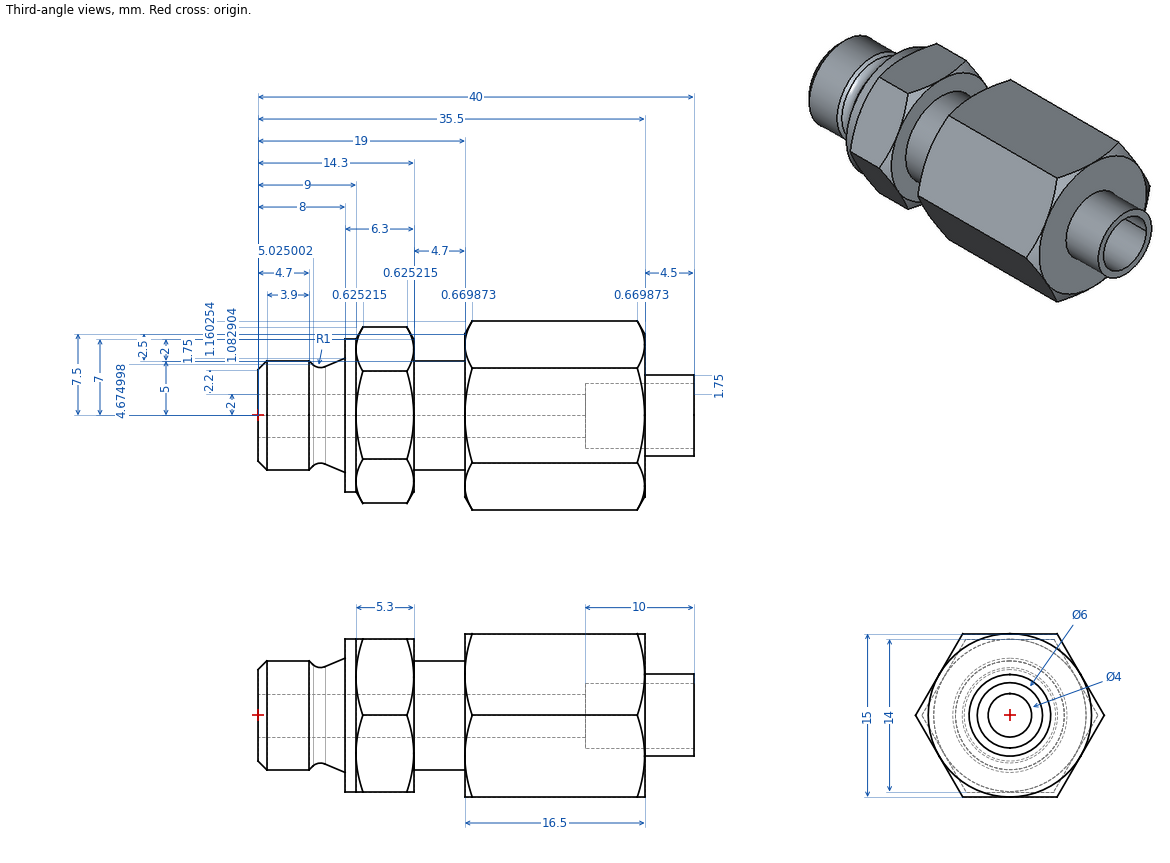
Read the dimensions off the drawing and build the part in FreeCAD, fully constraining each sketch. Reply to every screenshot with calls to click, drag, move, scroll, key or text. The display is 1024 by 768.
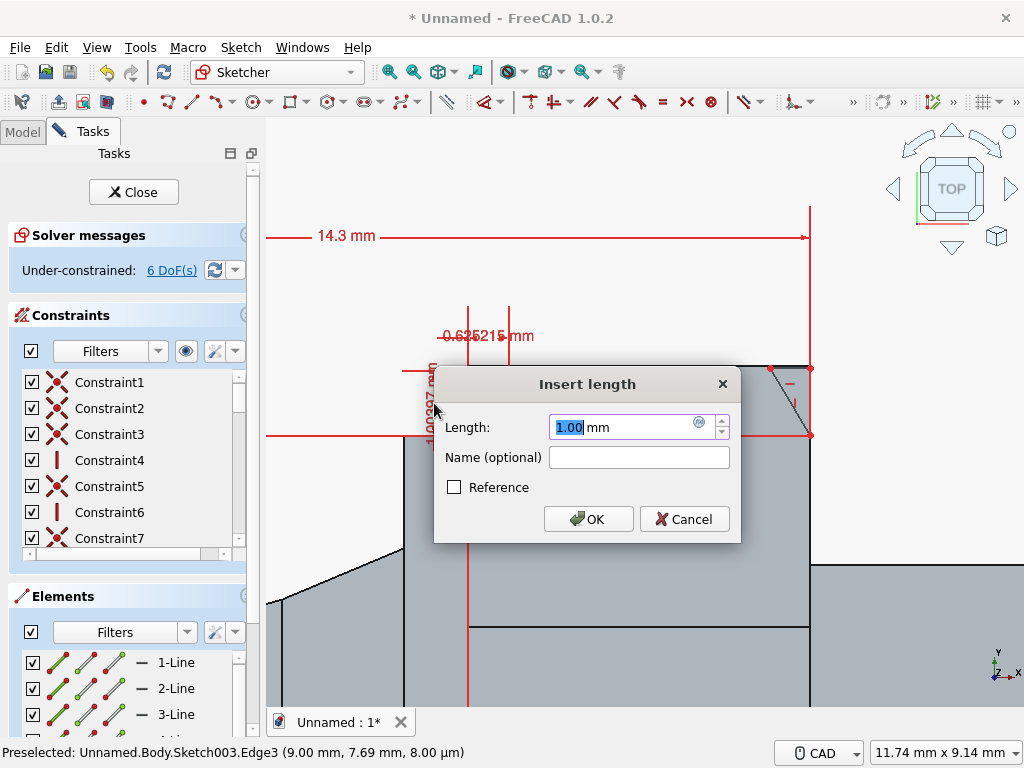
text(1.082904)
key(Return)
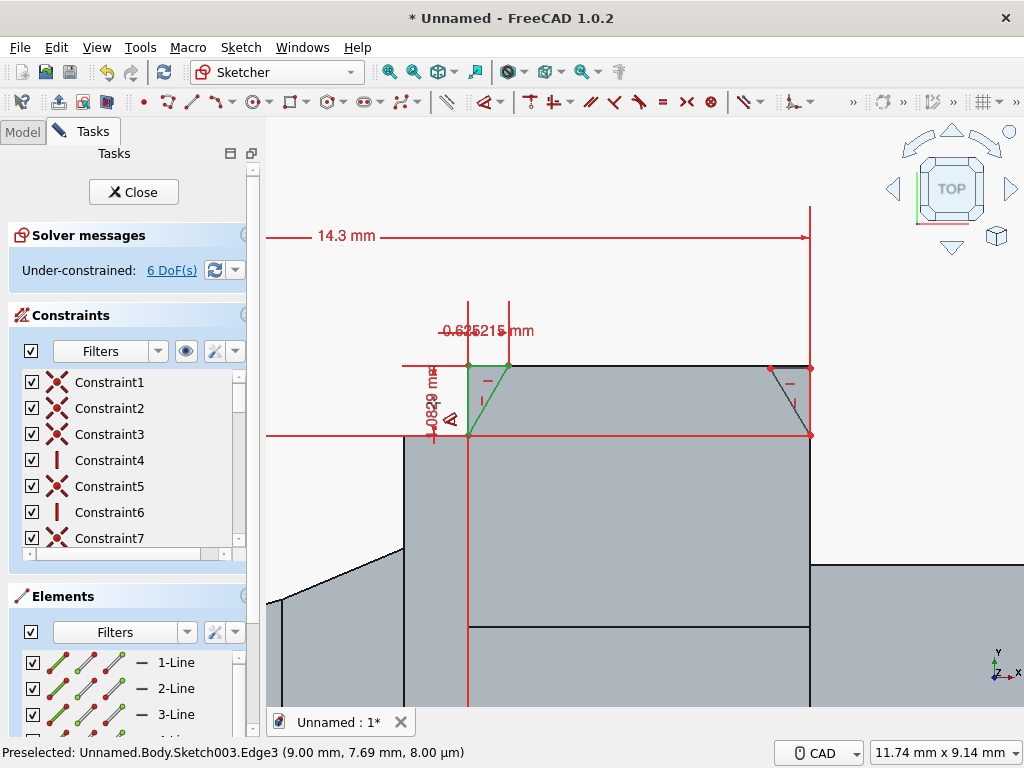
scroll(810, 415, up, 2)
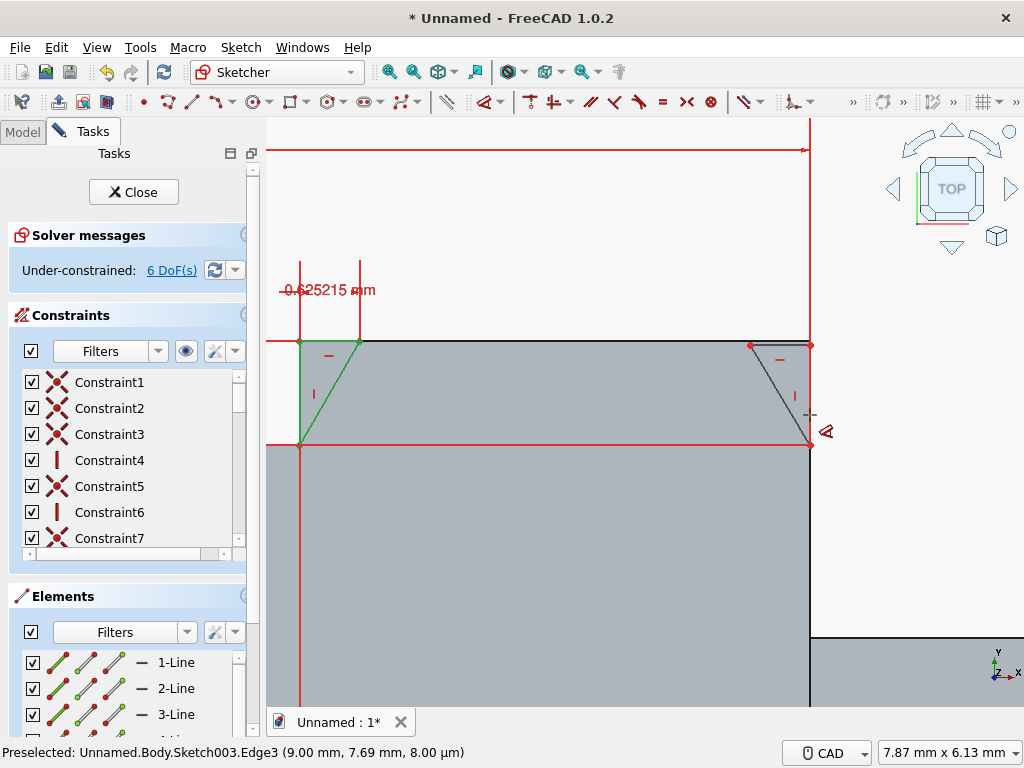
click(810, 415)
click(776, 418)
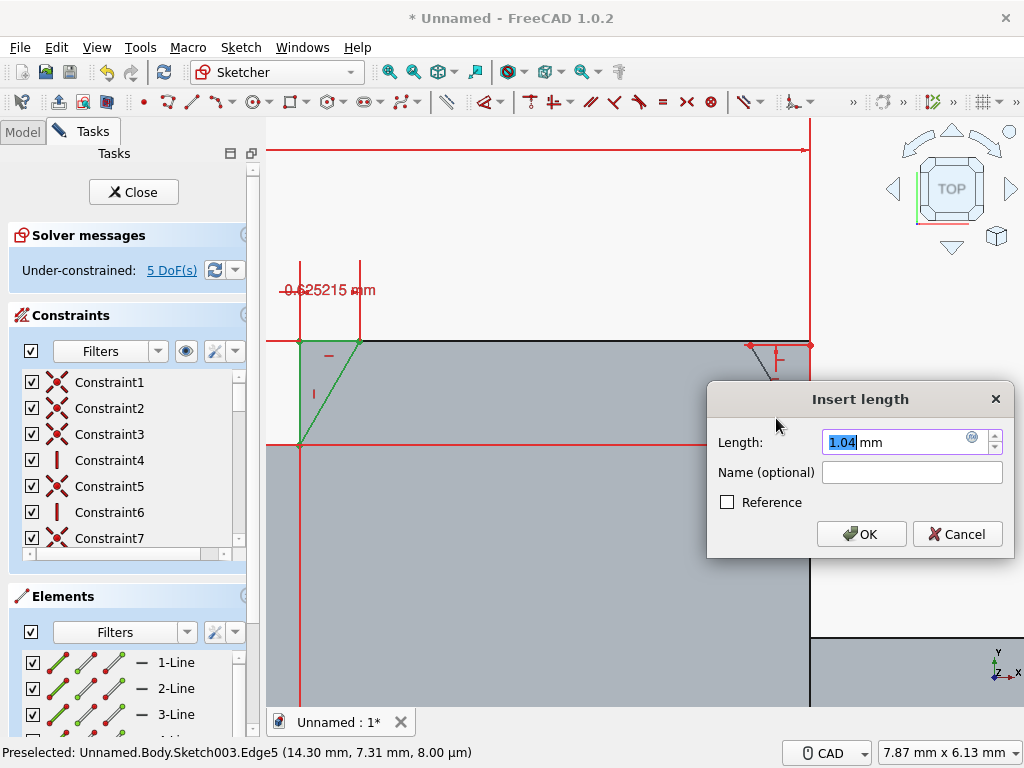
text(1.082904)
key(Return)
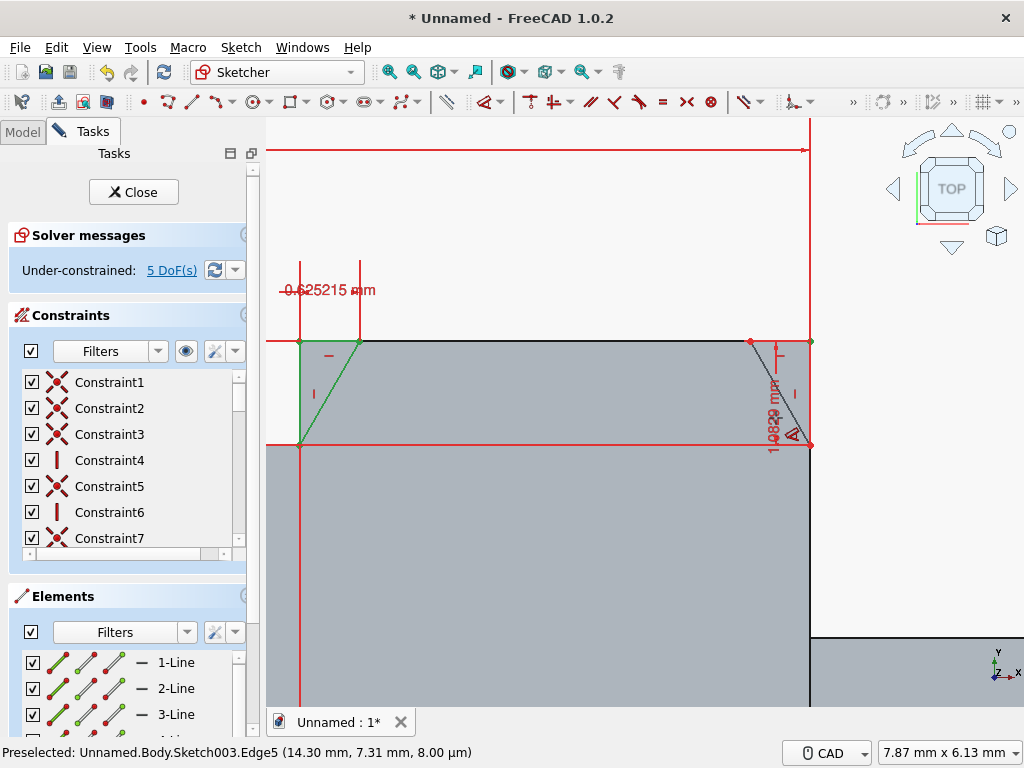
click(792, 341)
click(780, 307)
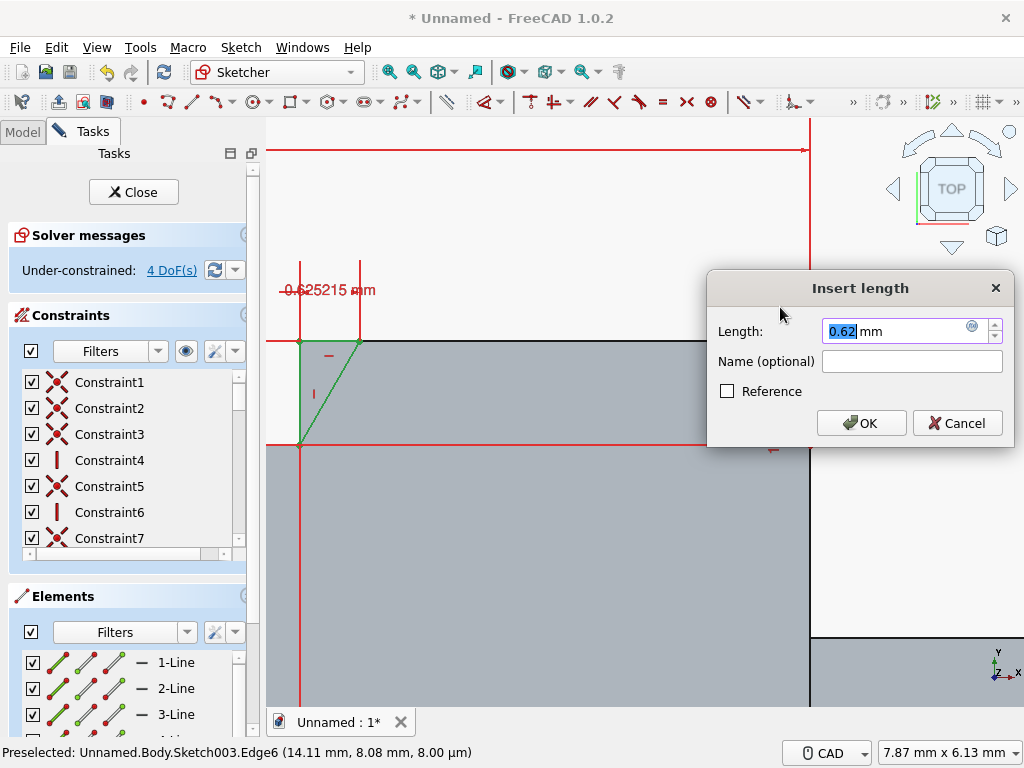
text(0.625215)
key(Return)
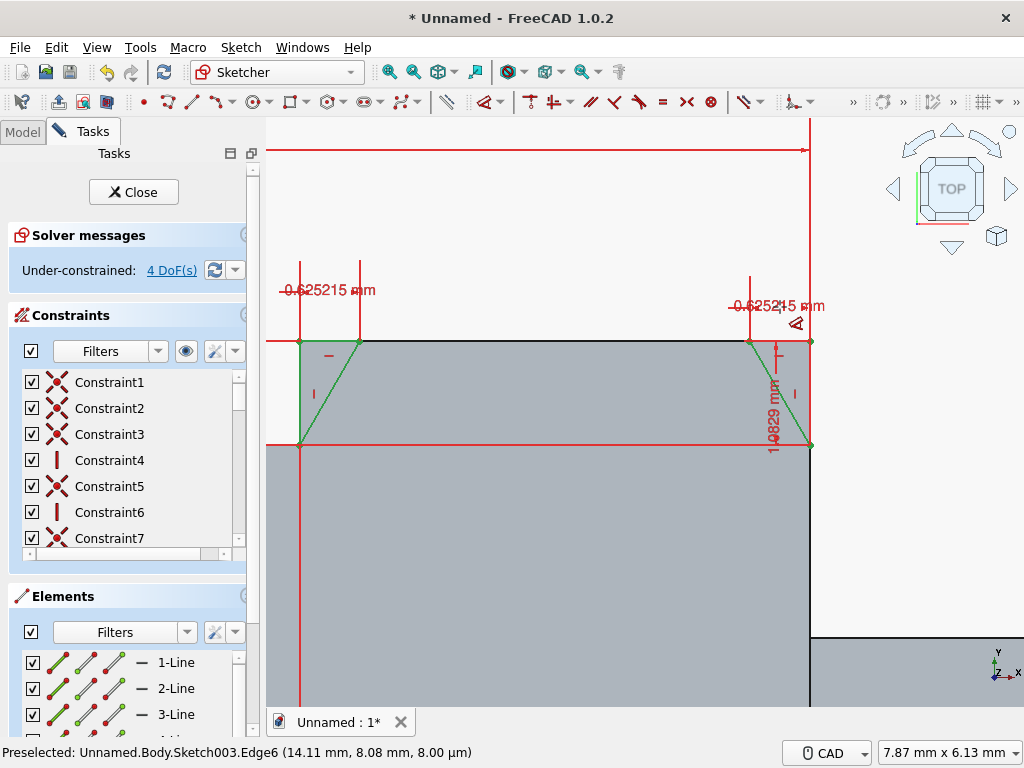
scroll(506, 376, down, 11)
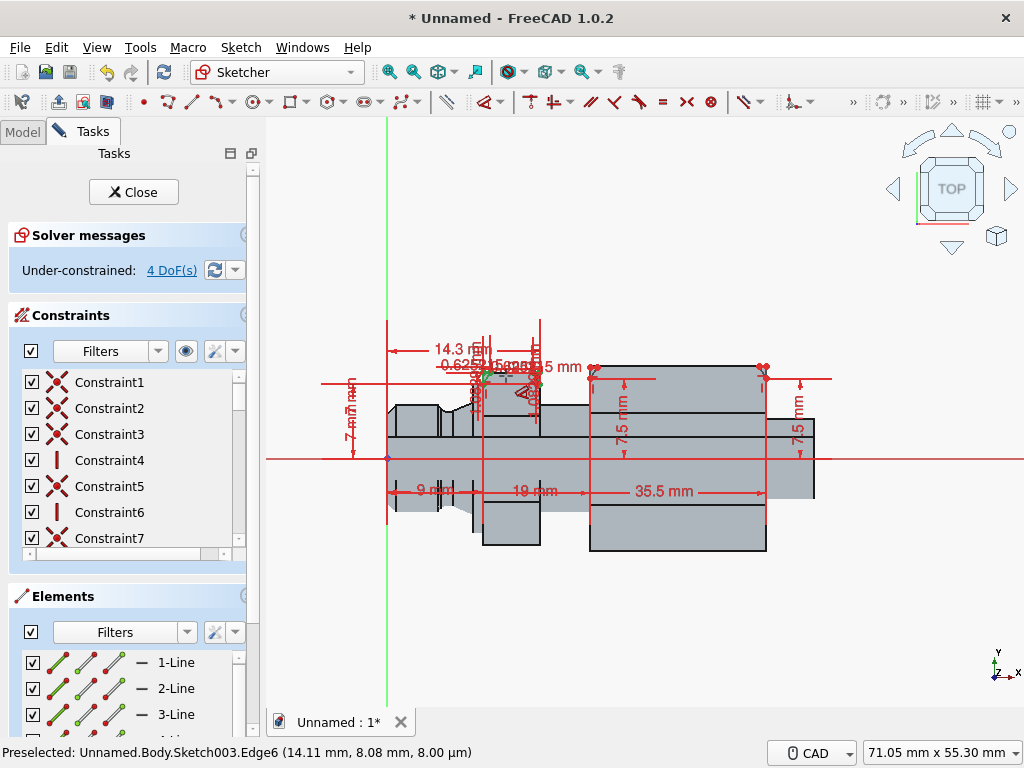
scroll(595, 367, up, 11)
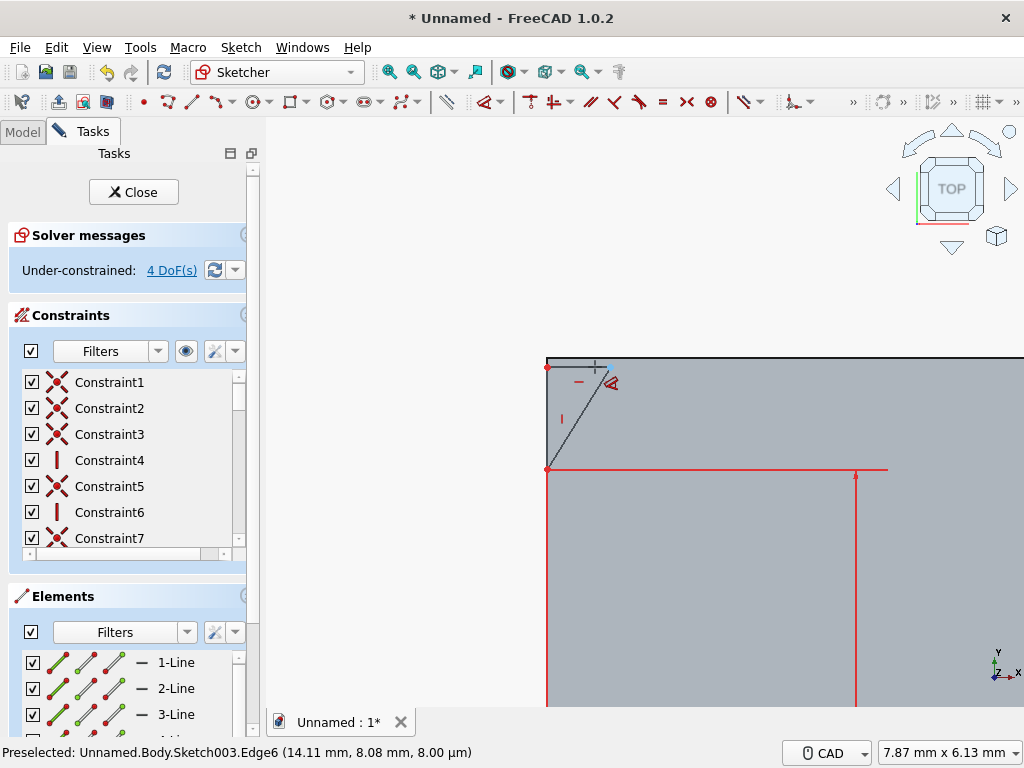
click(592, 367)
click(579, 333)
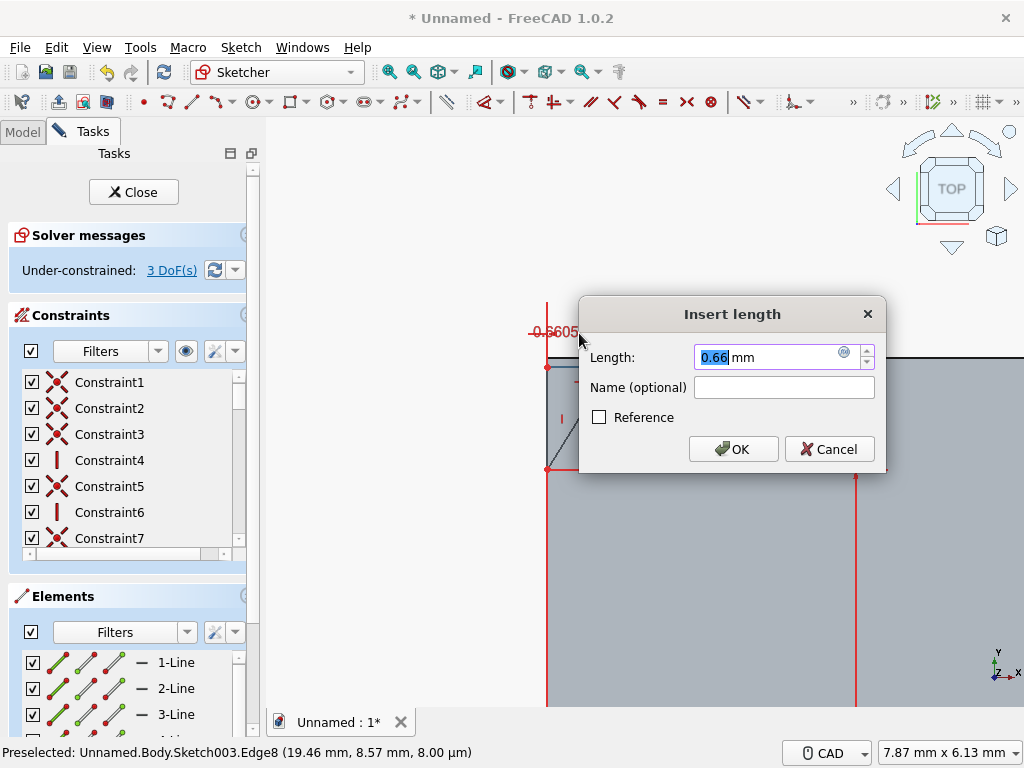
text(0.669873)
key(Return)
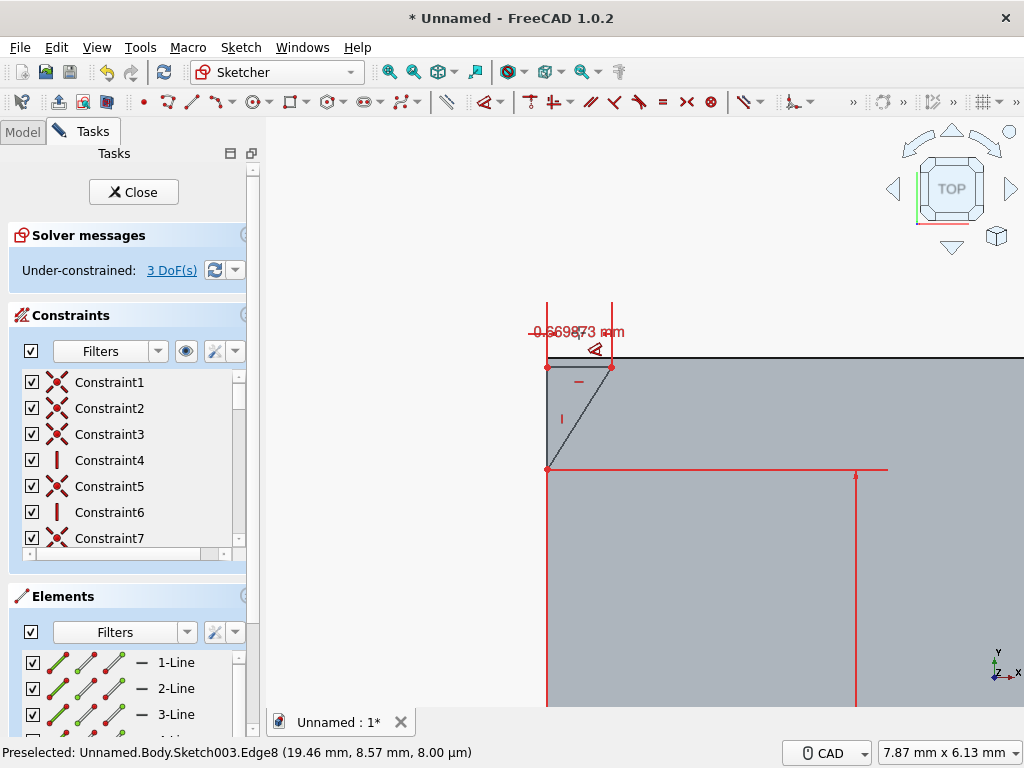
click(547, 398)
click(581, 442)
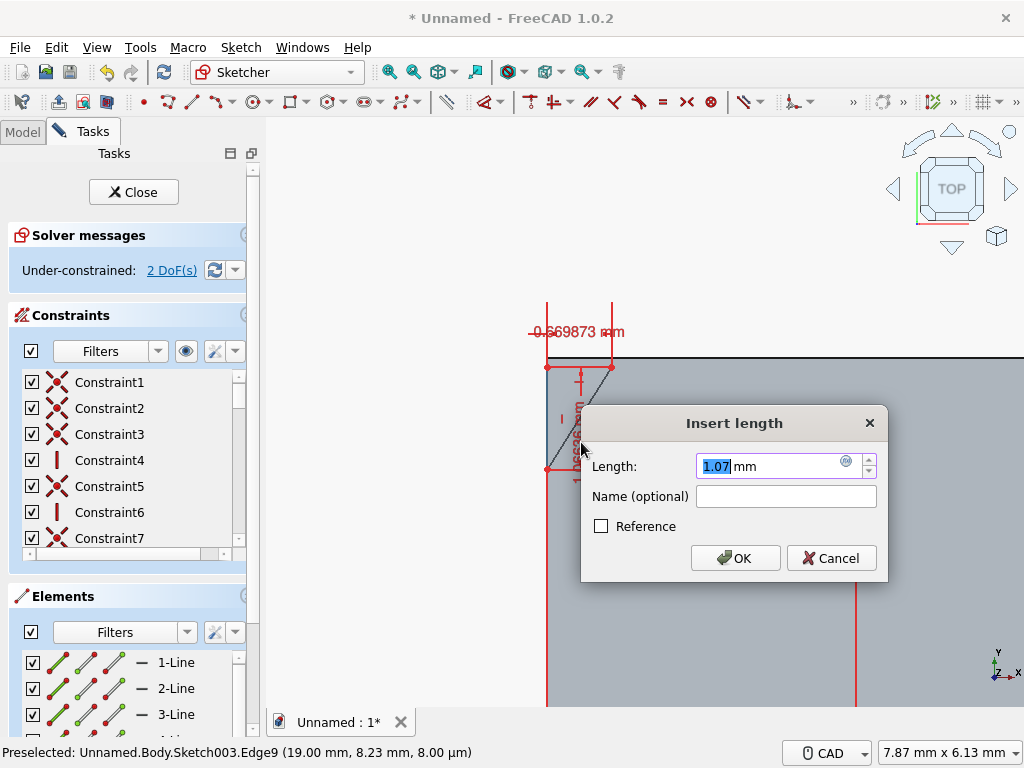
text(1.160254)
key(Return)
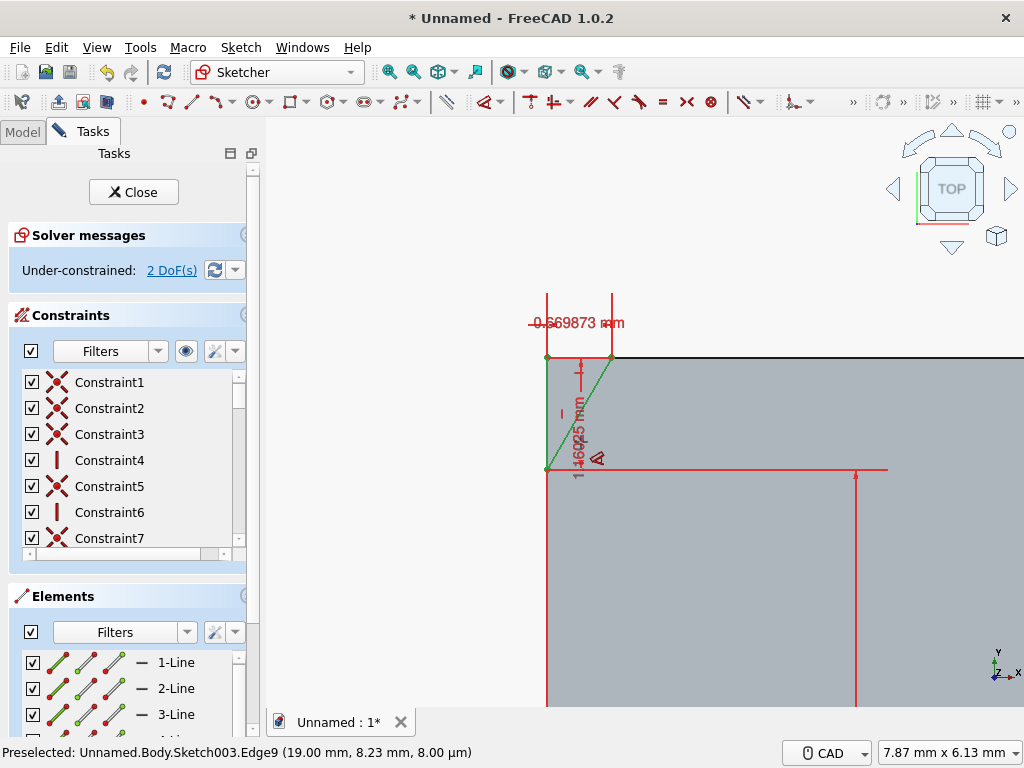
scroll(595, 367, down, 11)